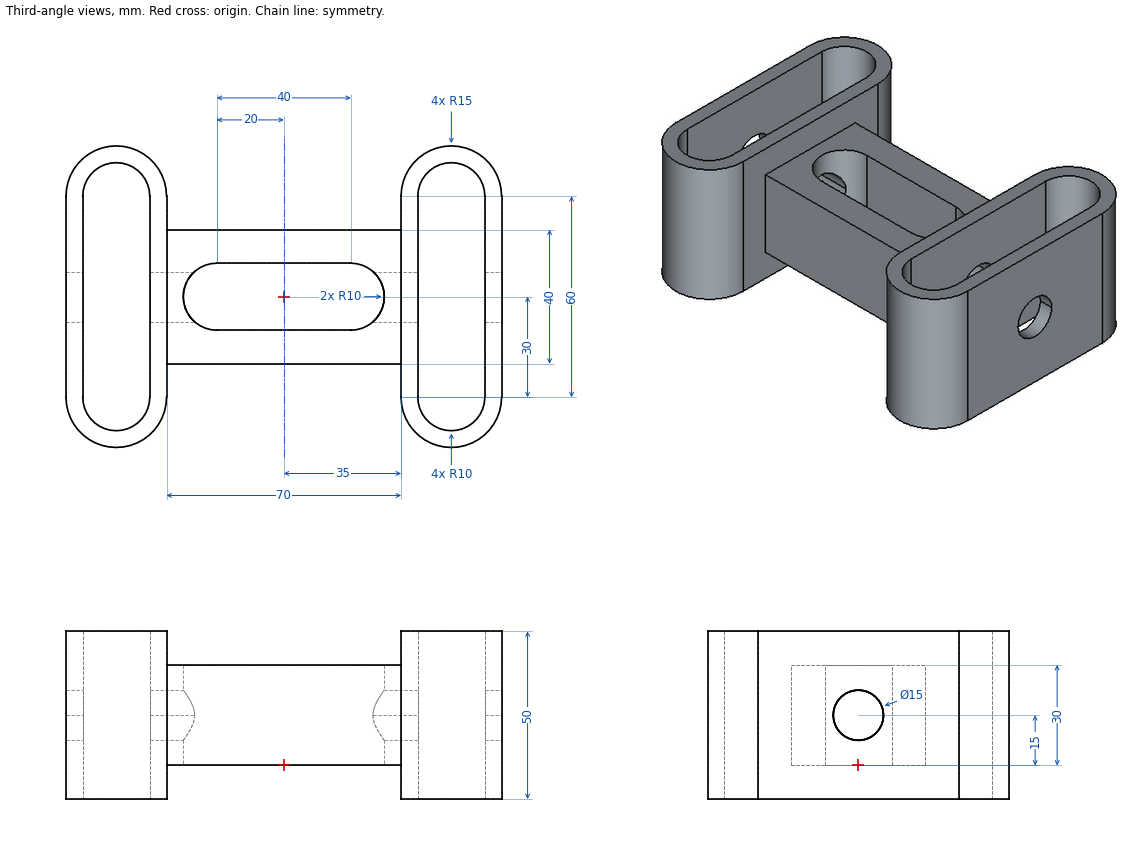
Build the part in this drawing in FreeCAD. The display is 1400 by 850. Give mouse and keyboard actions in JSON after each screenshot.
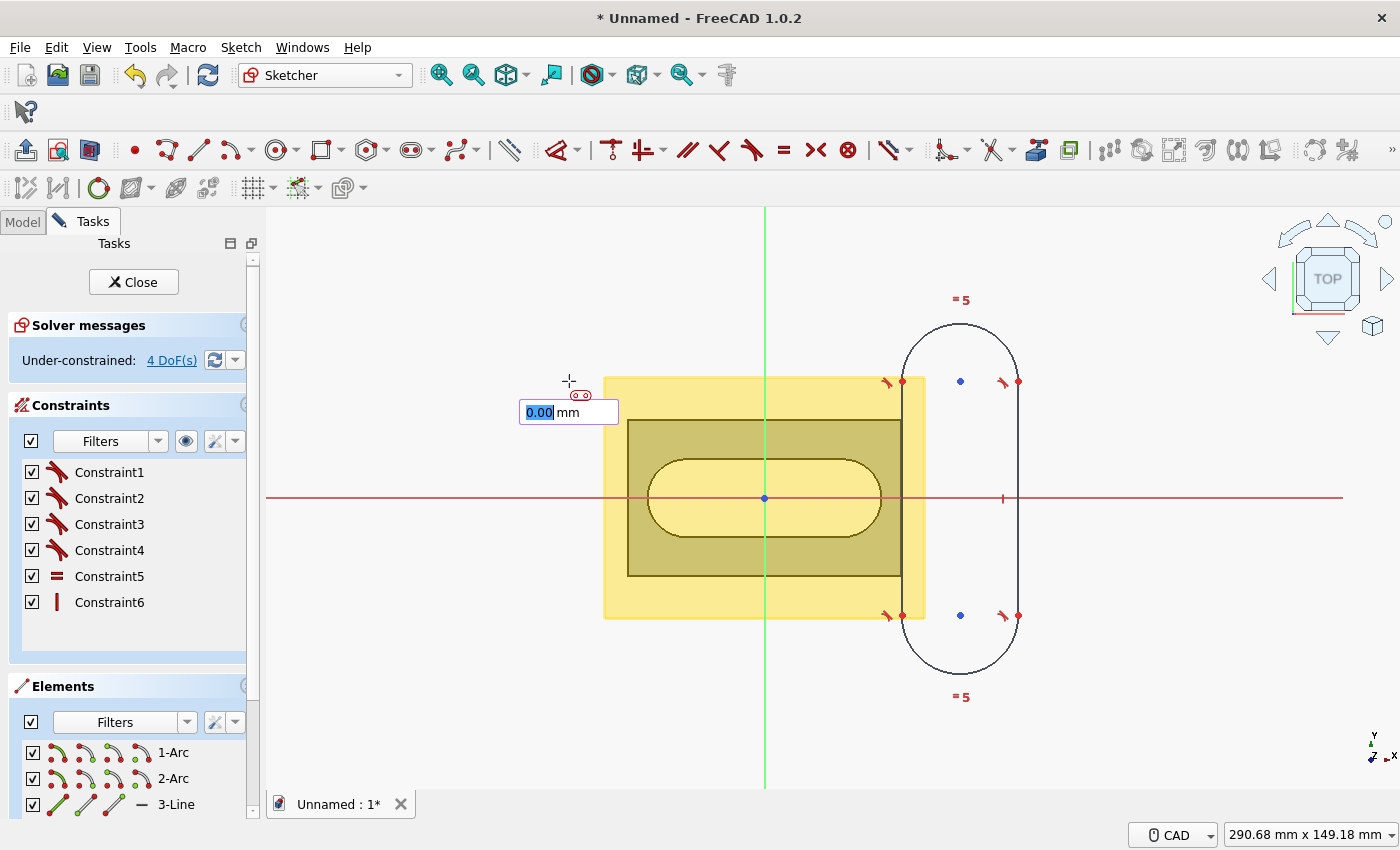
{"action": "left_click", "coordinate": [511, 463]}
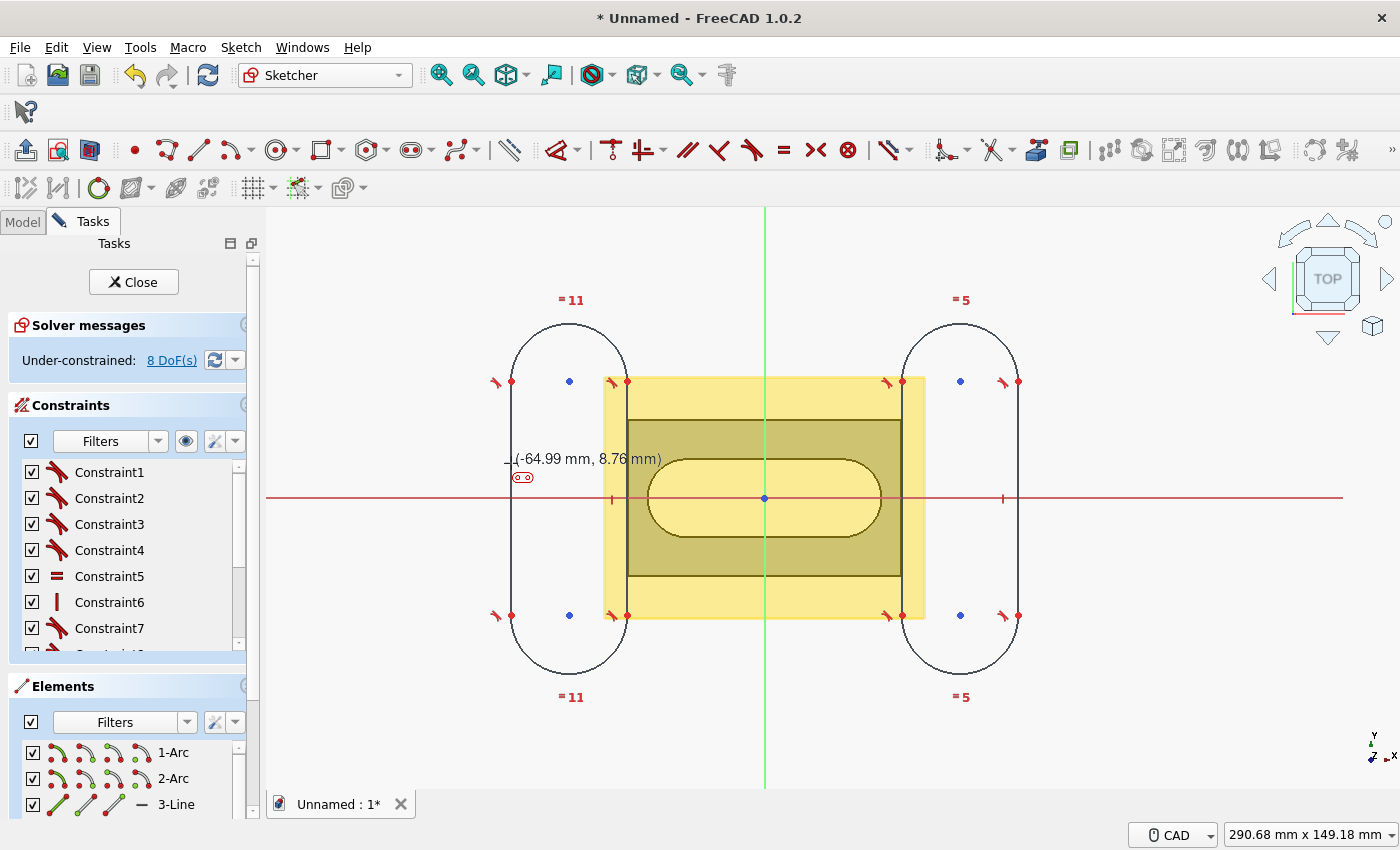
{"action": "left_click", "coordinate": [960, 616]}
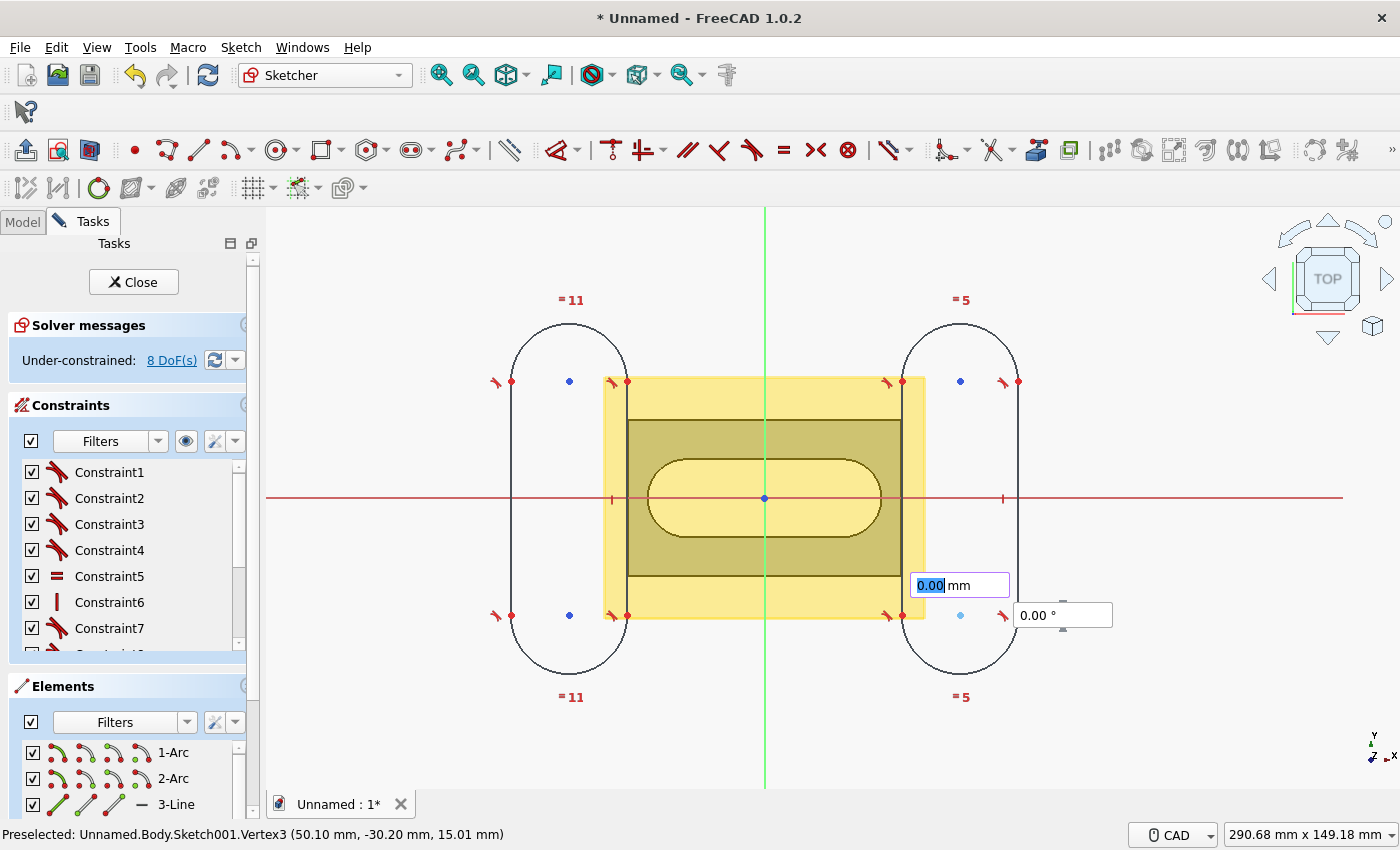
{"action": "left_click", "coordinate": [960, 382]}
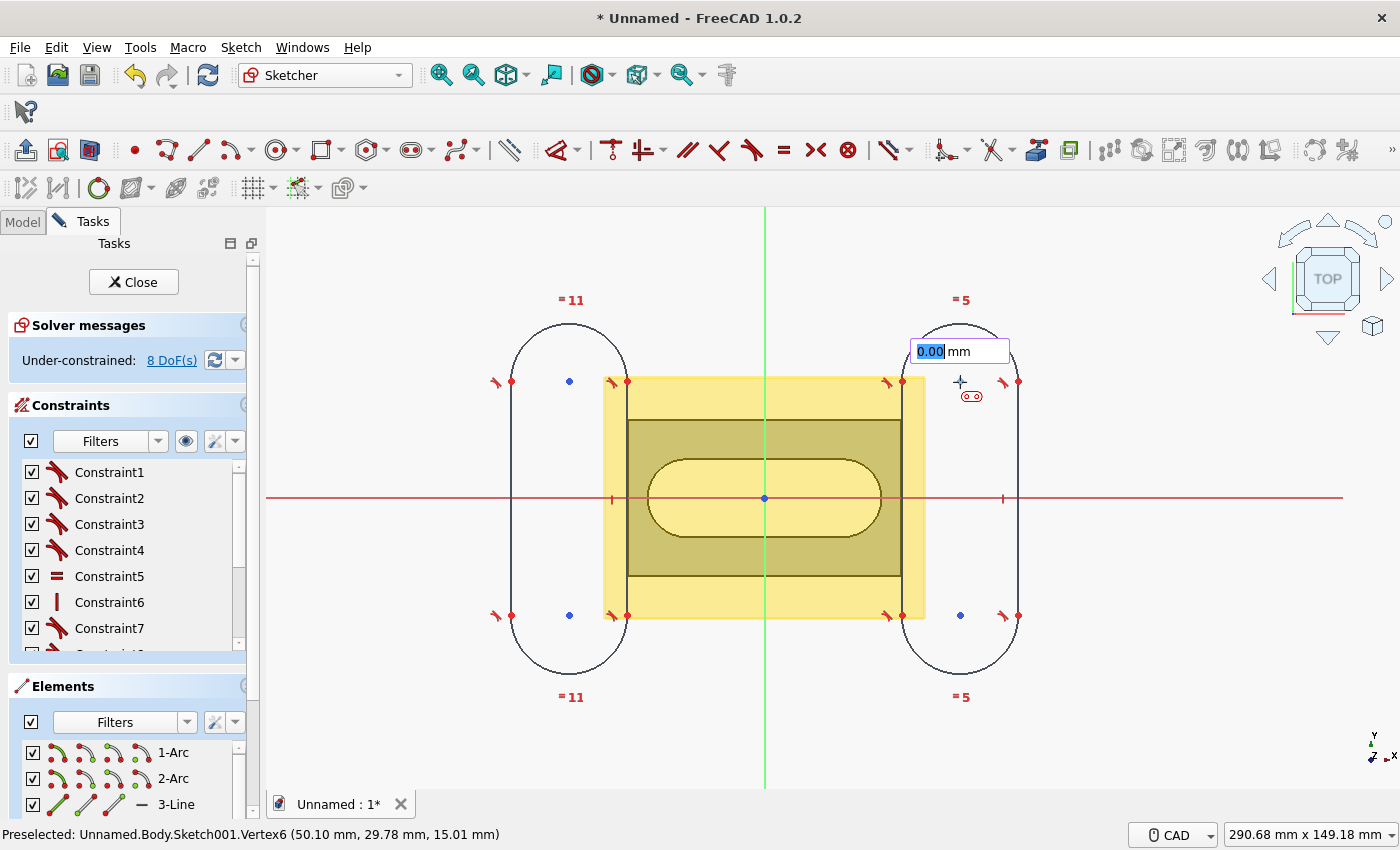
{"action": "left_click", "coordinate": [999, 463]}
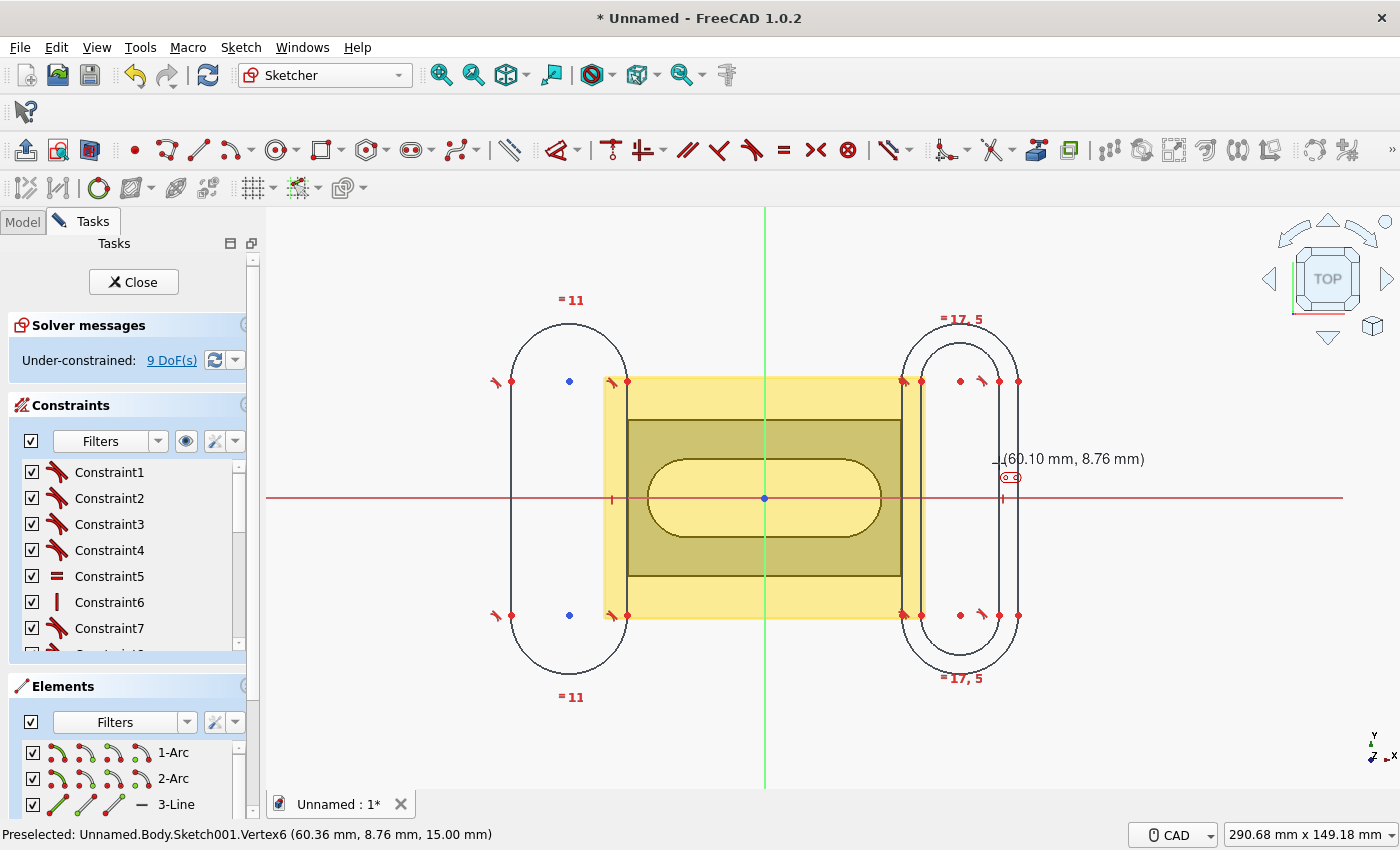
{"action": "left_click", "coordinate": [569, 616]}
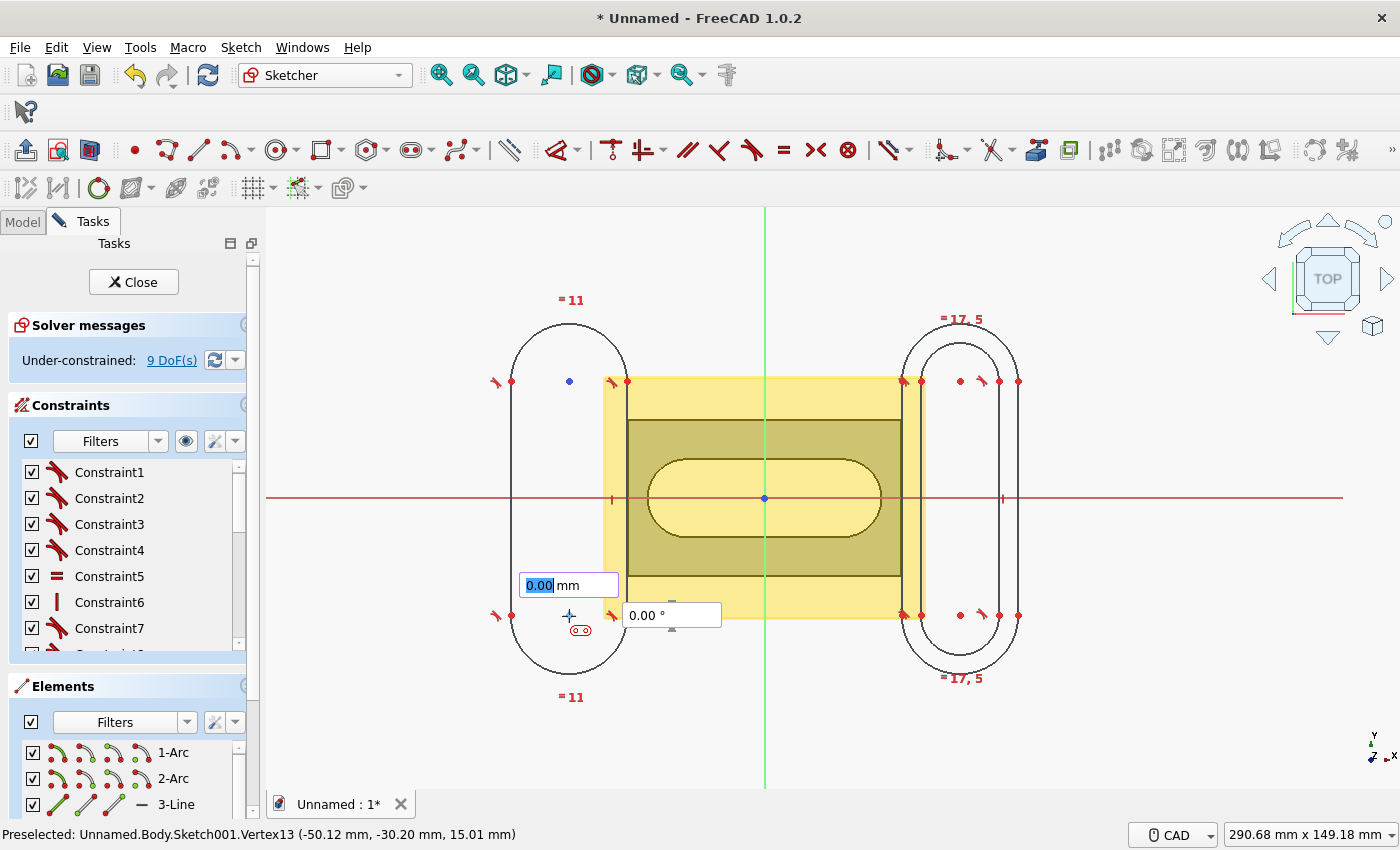
{"action": "left_click", "coordinate": [569, 382]}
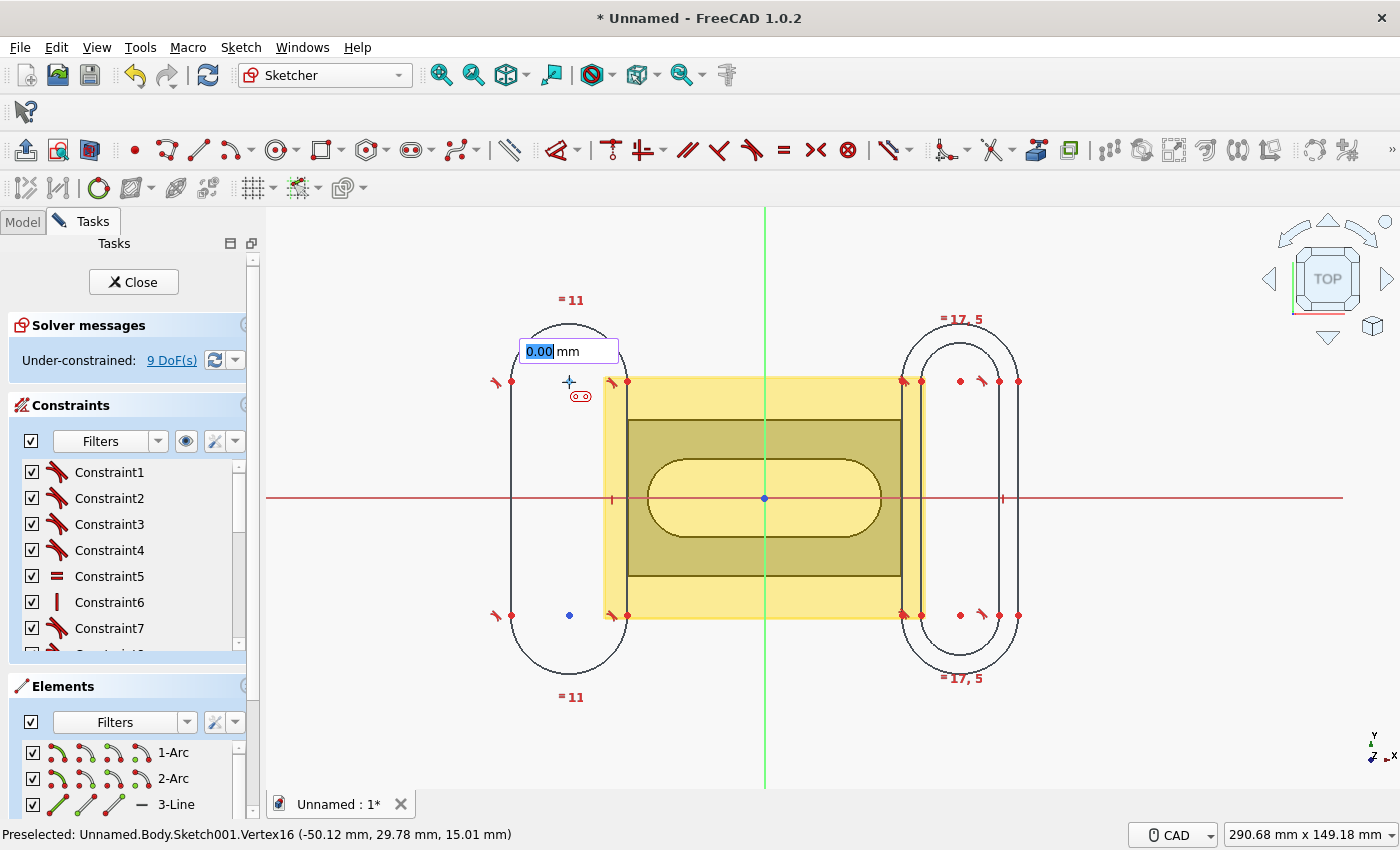
{"action": "left_click", "coordinate": [608, 463]}
{"action": "key", "text": "Escape"}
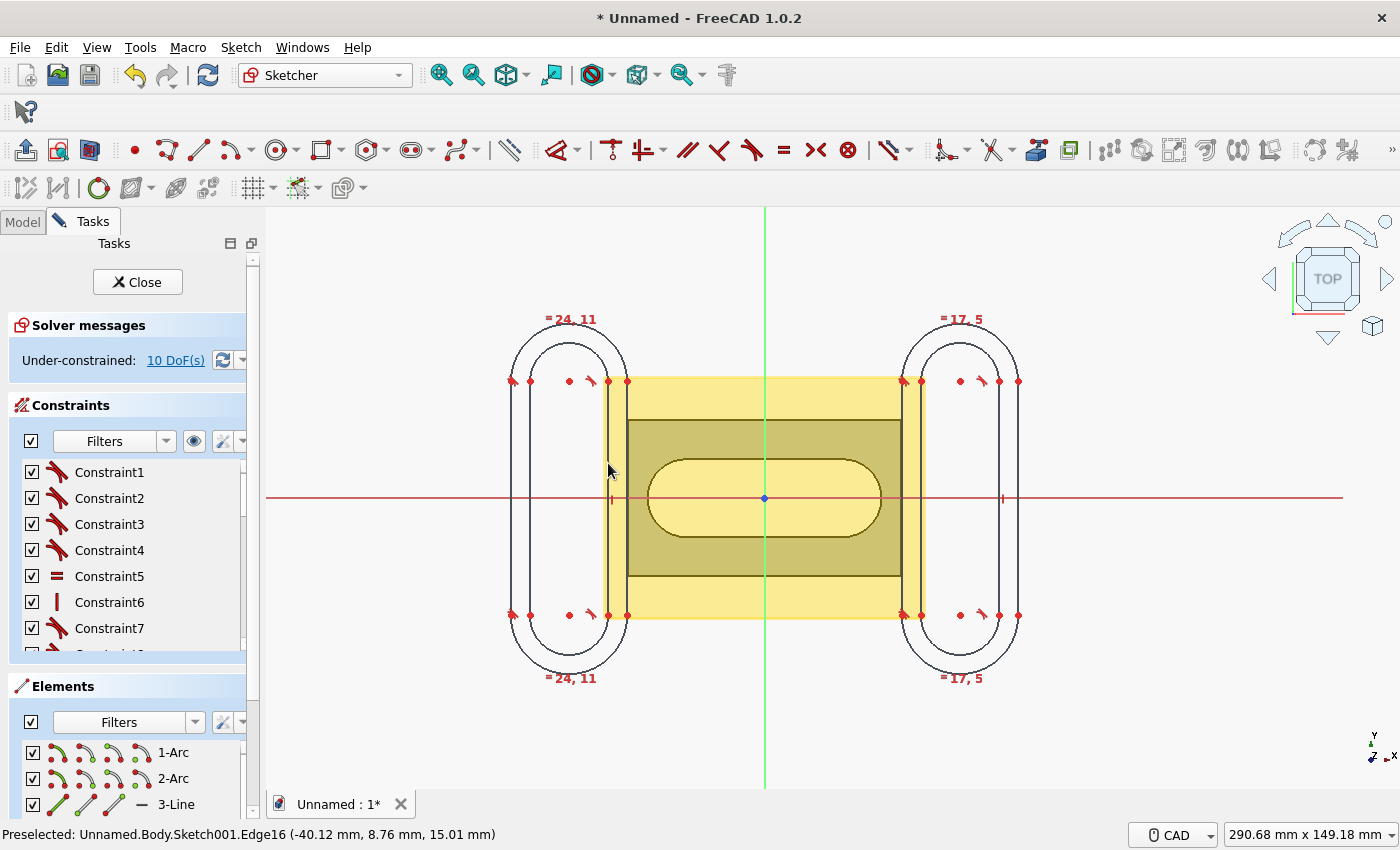
{"action": "left_click", "coordinate": [926, 663]}